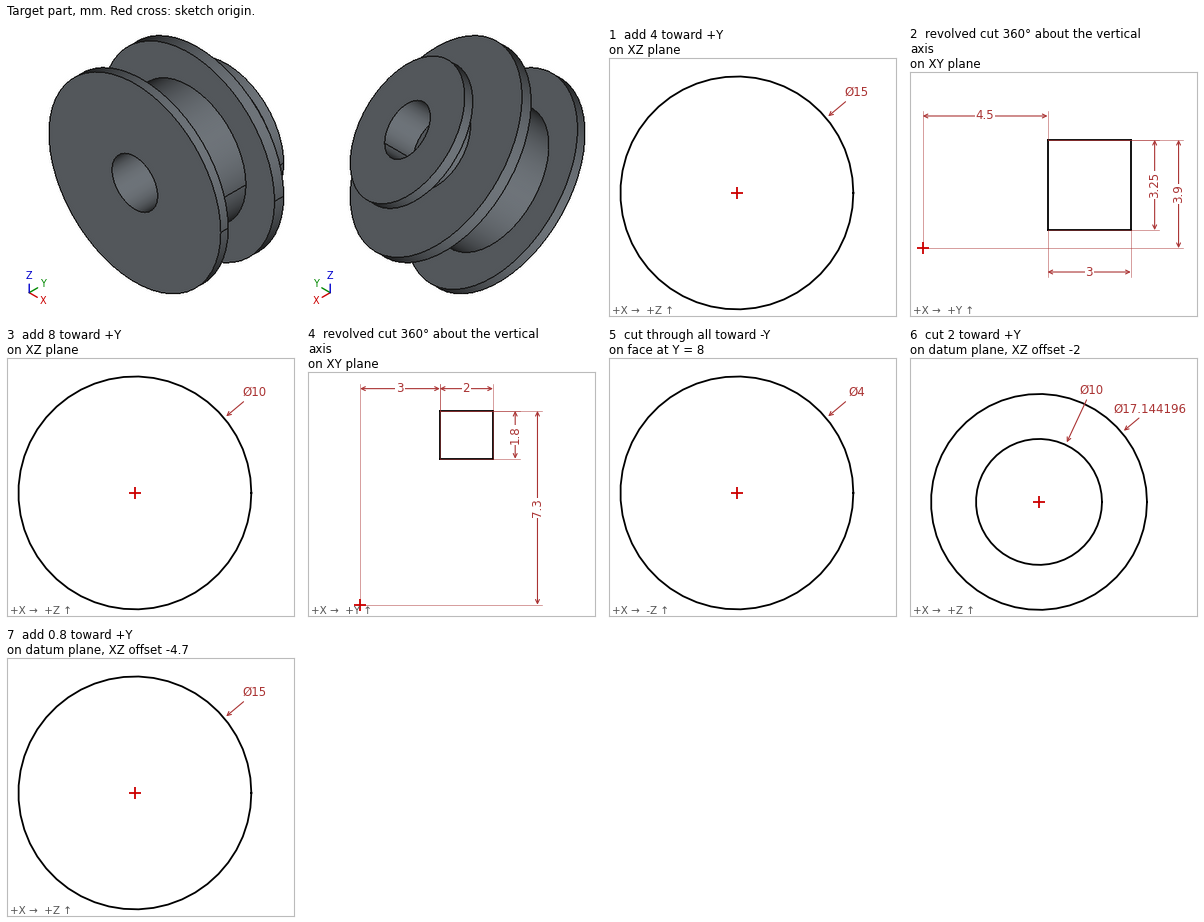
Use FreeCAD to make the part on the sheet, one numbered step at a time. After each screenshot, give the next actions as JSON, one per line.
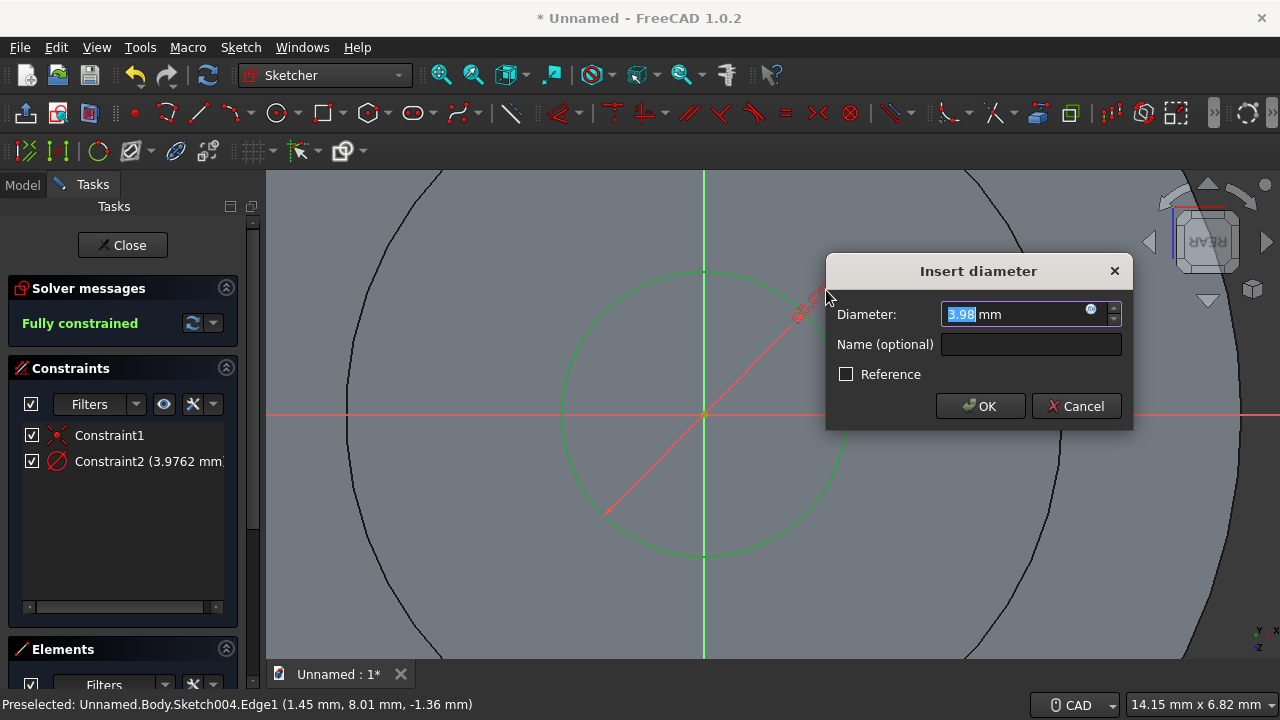
{"action": "type", "text": "4"}
{"action": "key", "text": "Return"}
{"action": "key", "text": "Escape"}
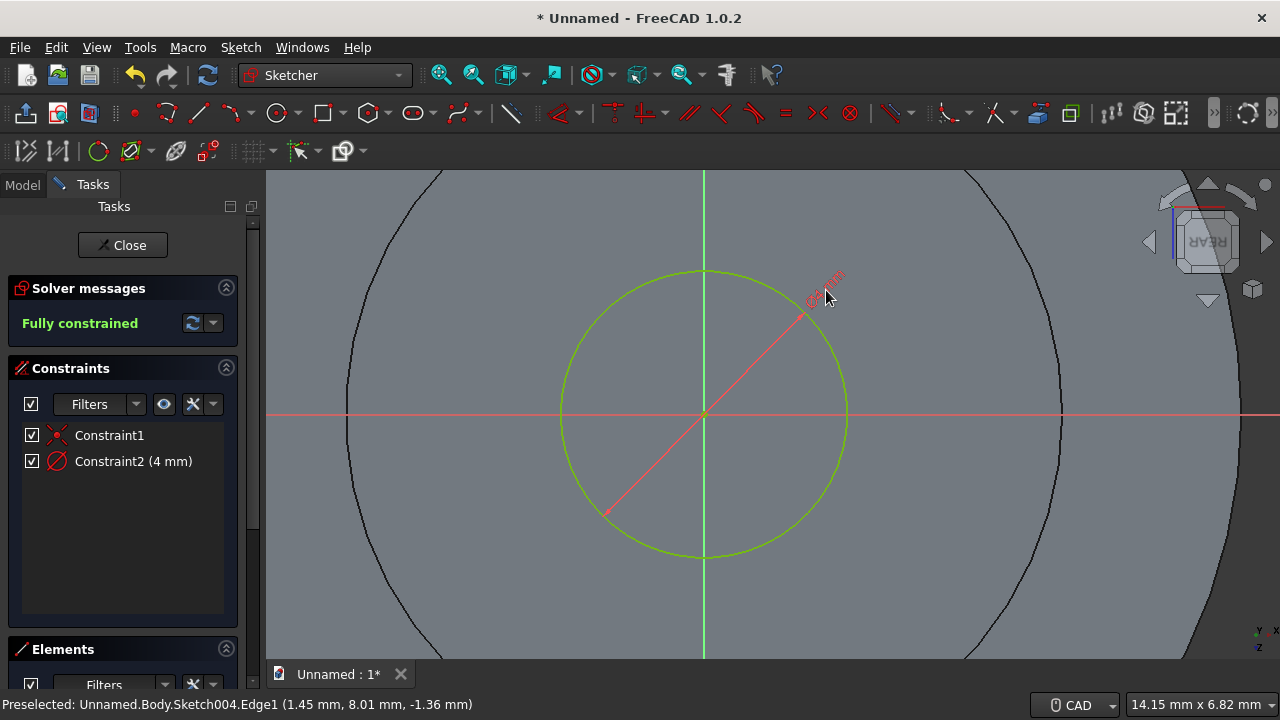
{"action": "left_click", "coordinate": [123, 245]}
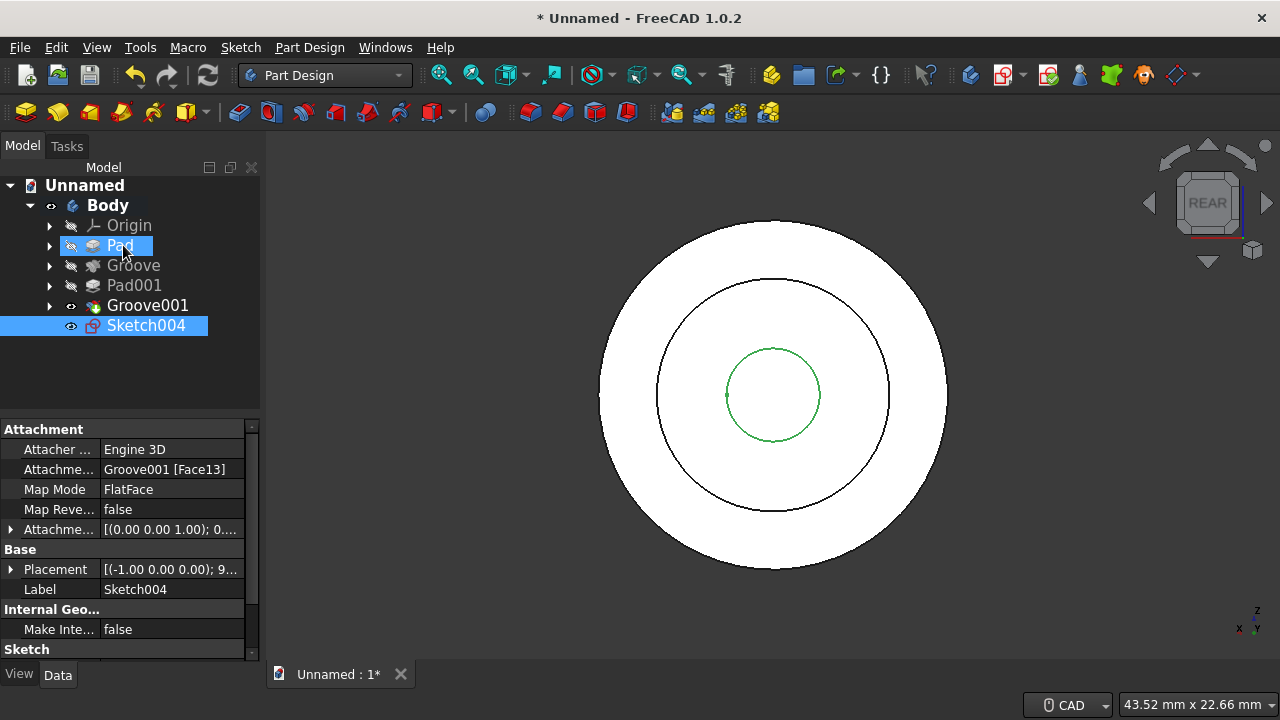
{"action": "left_click", "coordinate": [240, 112]}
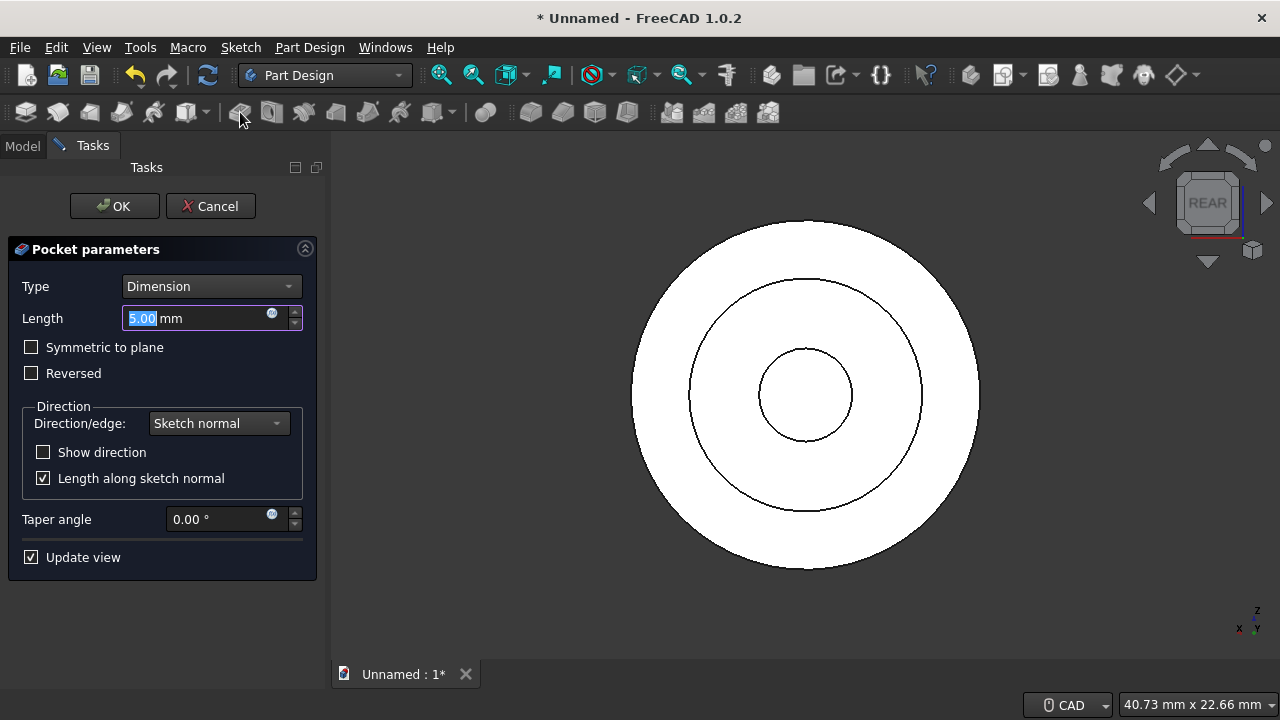
{"action": "left_click", "coordinate": [212, 286]}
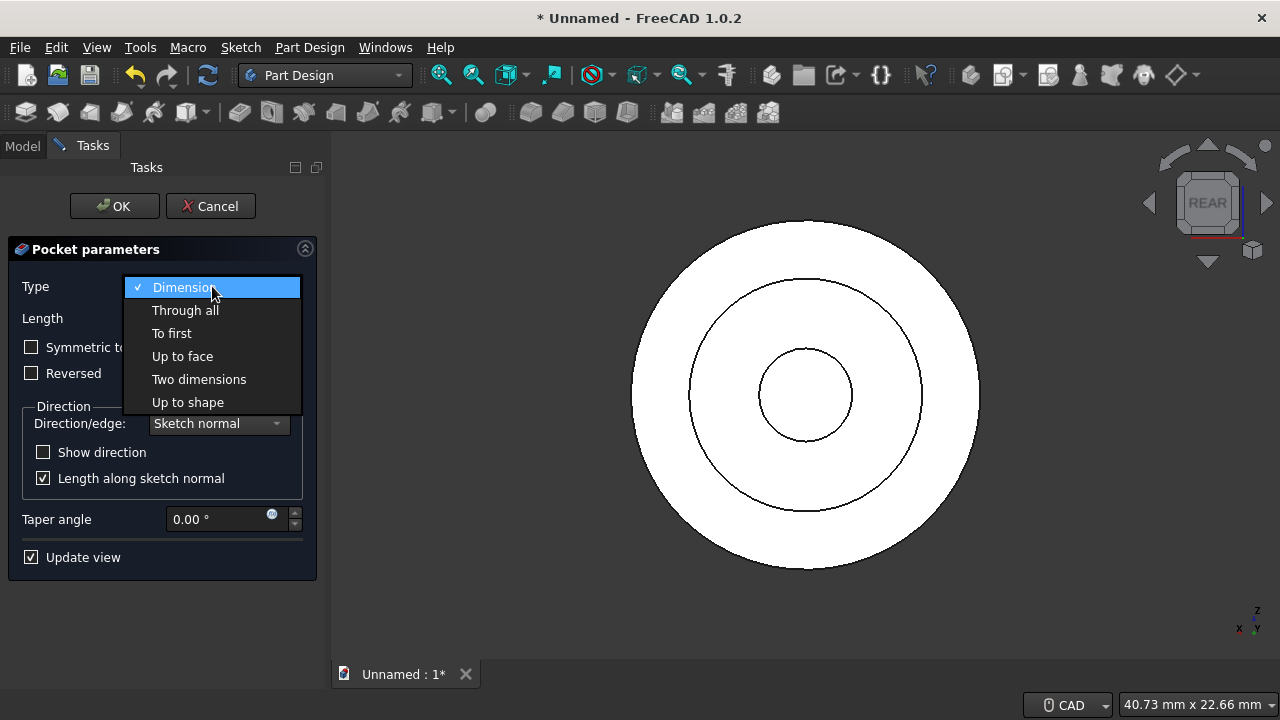
{"action": "left_click", "coordinate": [212, 310]}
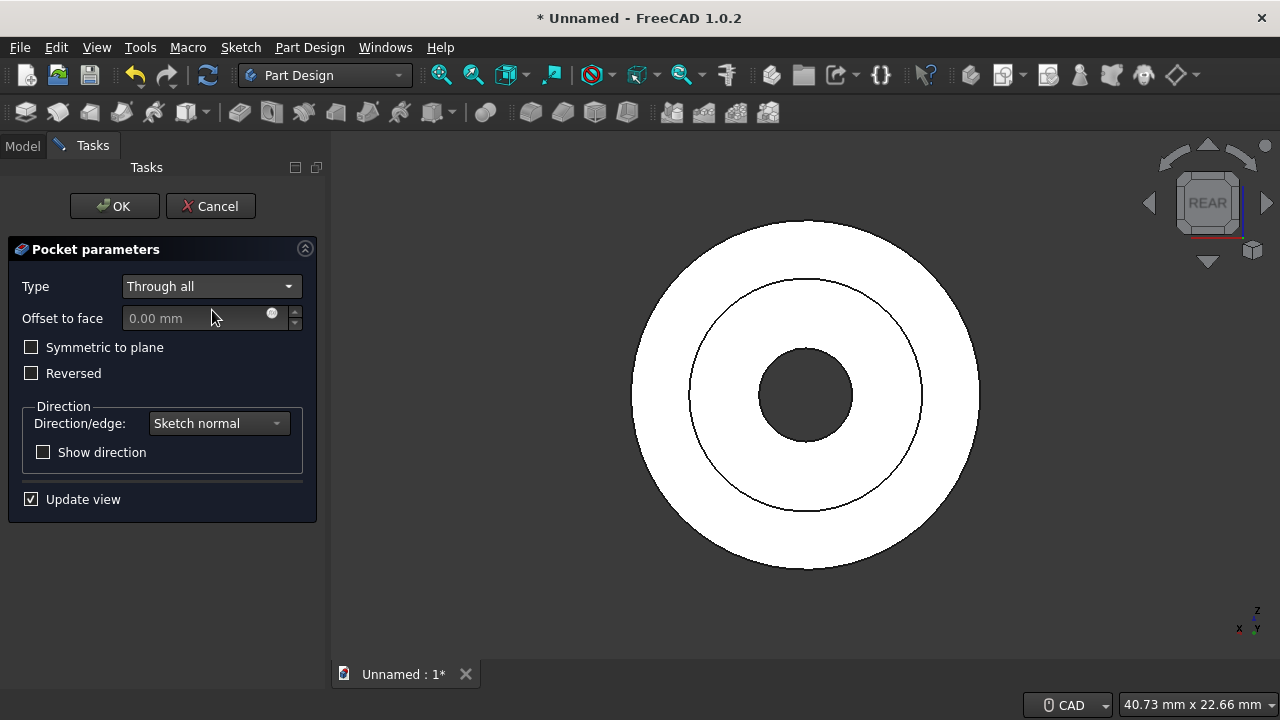
{"action": "left_click", "coordinate": [115, 206]}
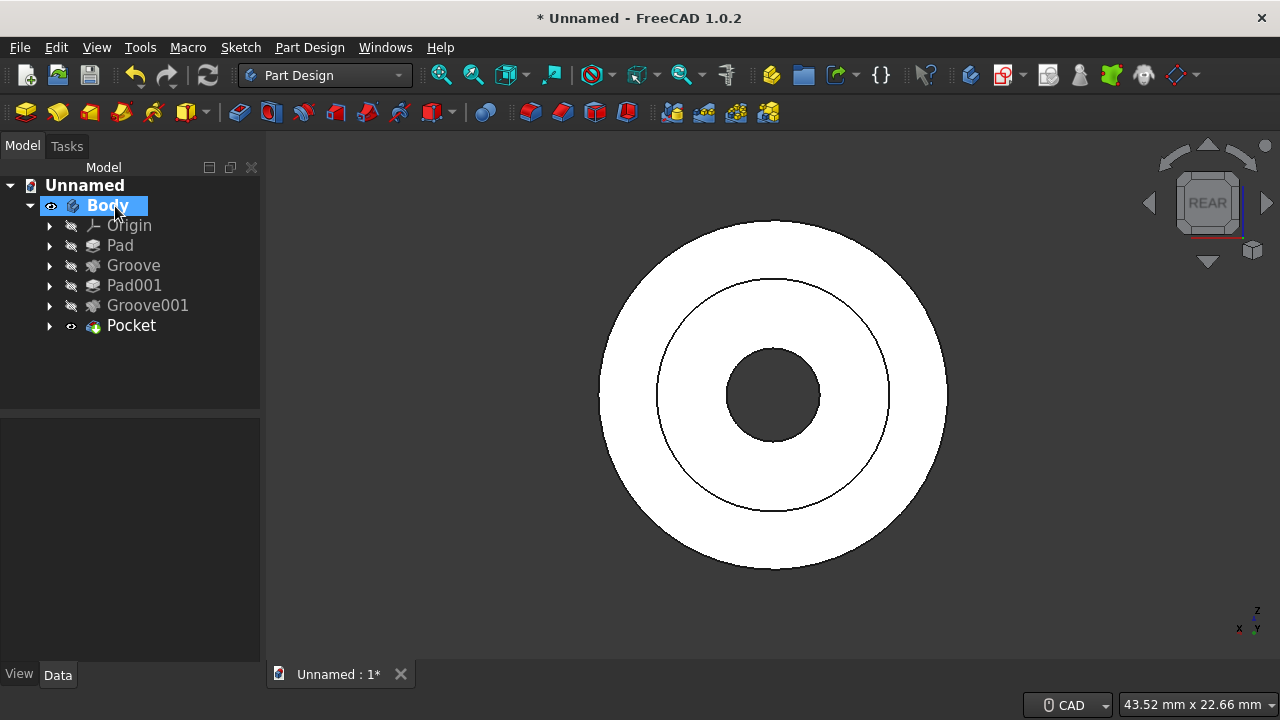
{"action": "left_click", "coordinate": [50, 226]}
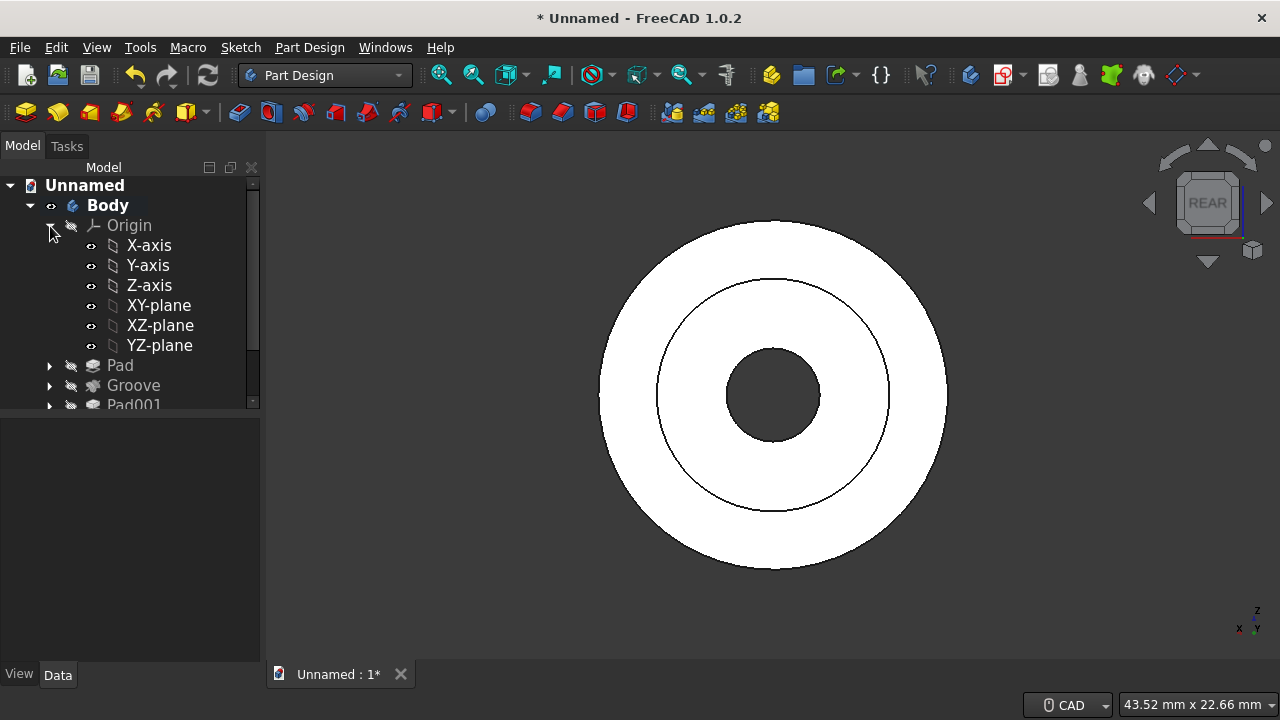
{"action": "left_click", "coordinate": [136, 326]}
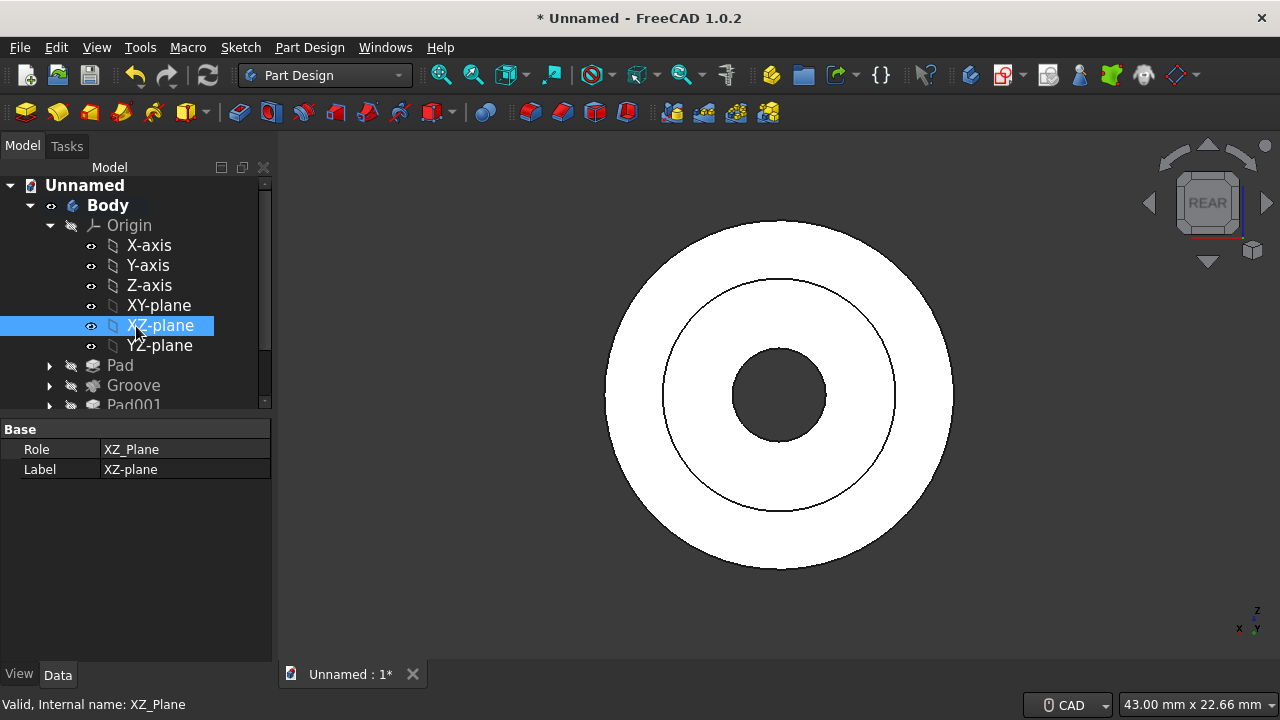
{"action": "left_click", "coordinate": [1176, 76]}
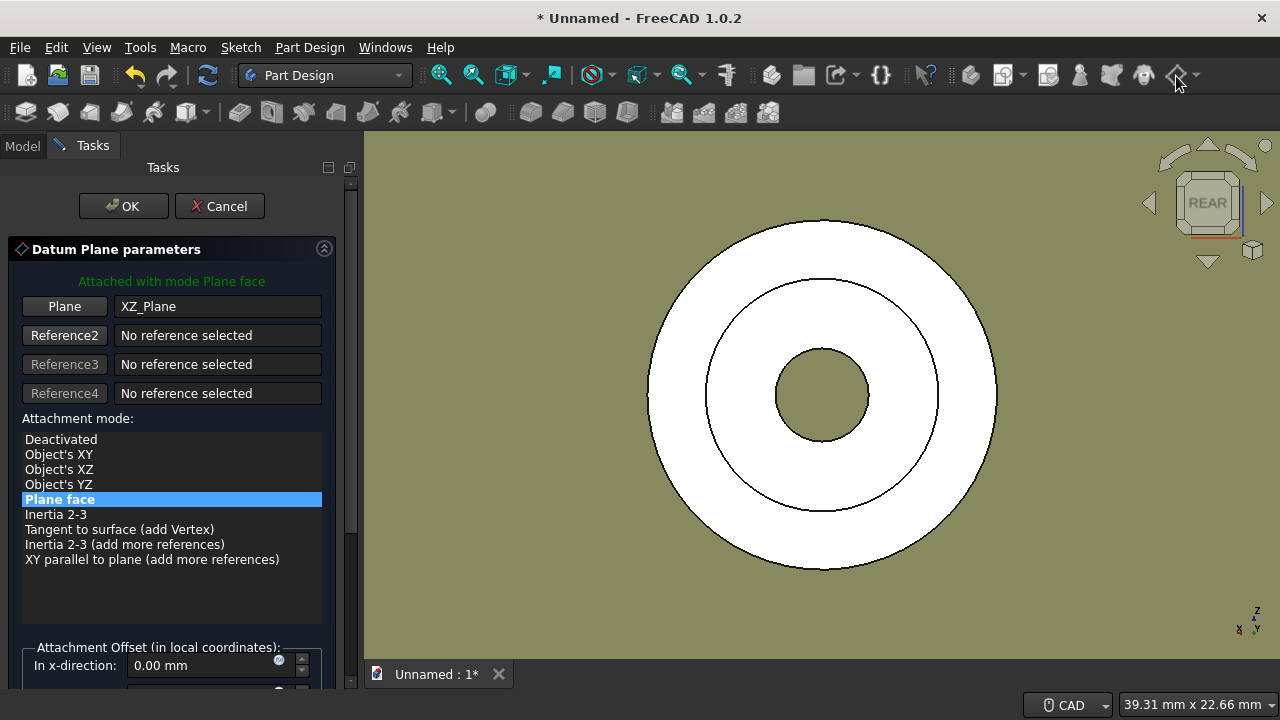
{"action": "scroll", "coordinate": [351, 432], "scroll_direction": "down", "scroll_amount": 2}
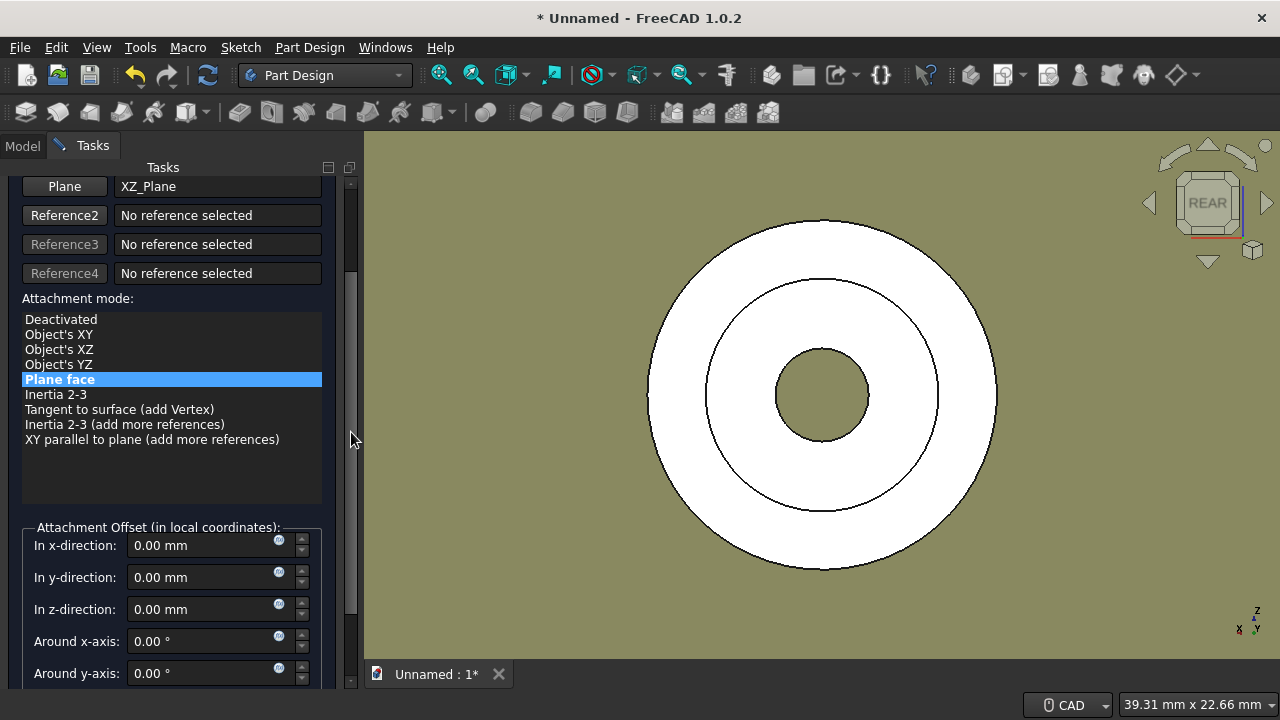
{"action": "triple_click", "coordinate": [210, 609]}